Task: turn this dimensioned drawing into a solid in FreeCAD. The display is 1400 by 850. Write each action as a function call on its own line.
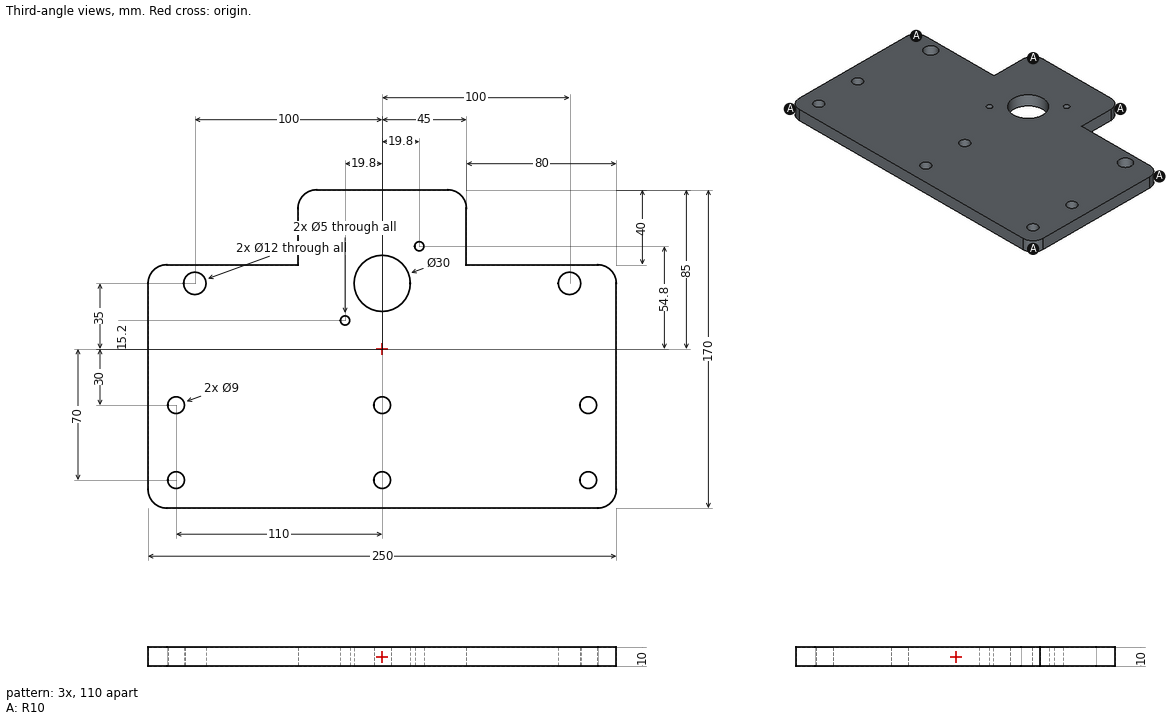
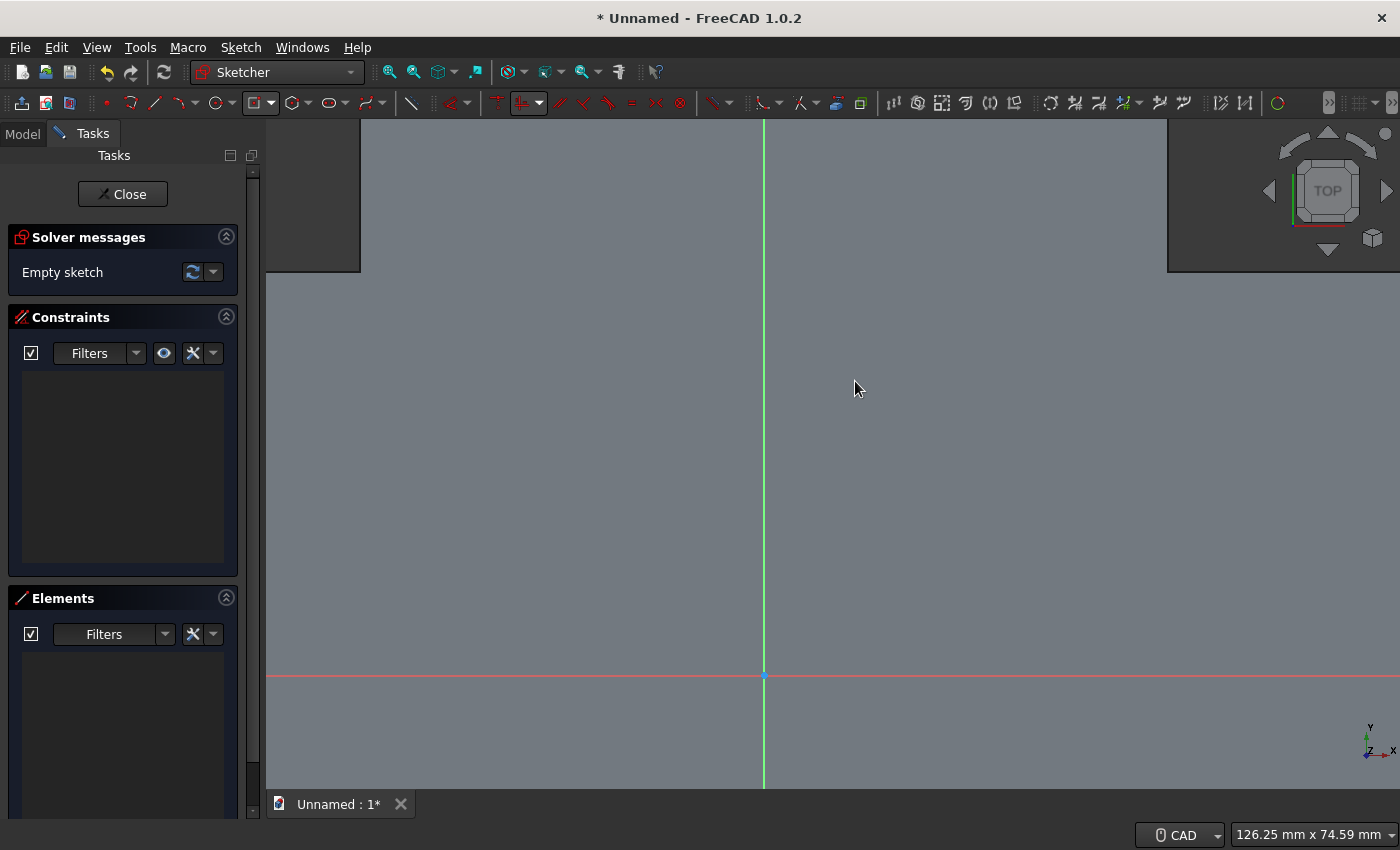
click(216, 104)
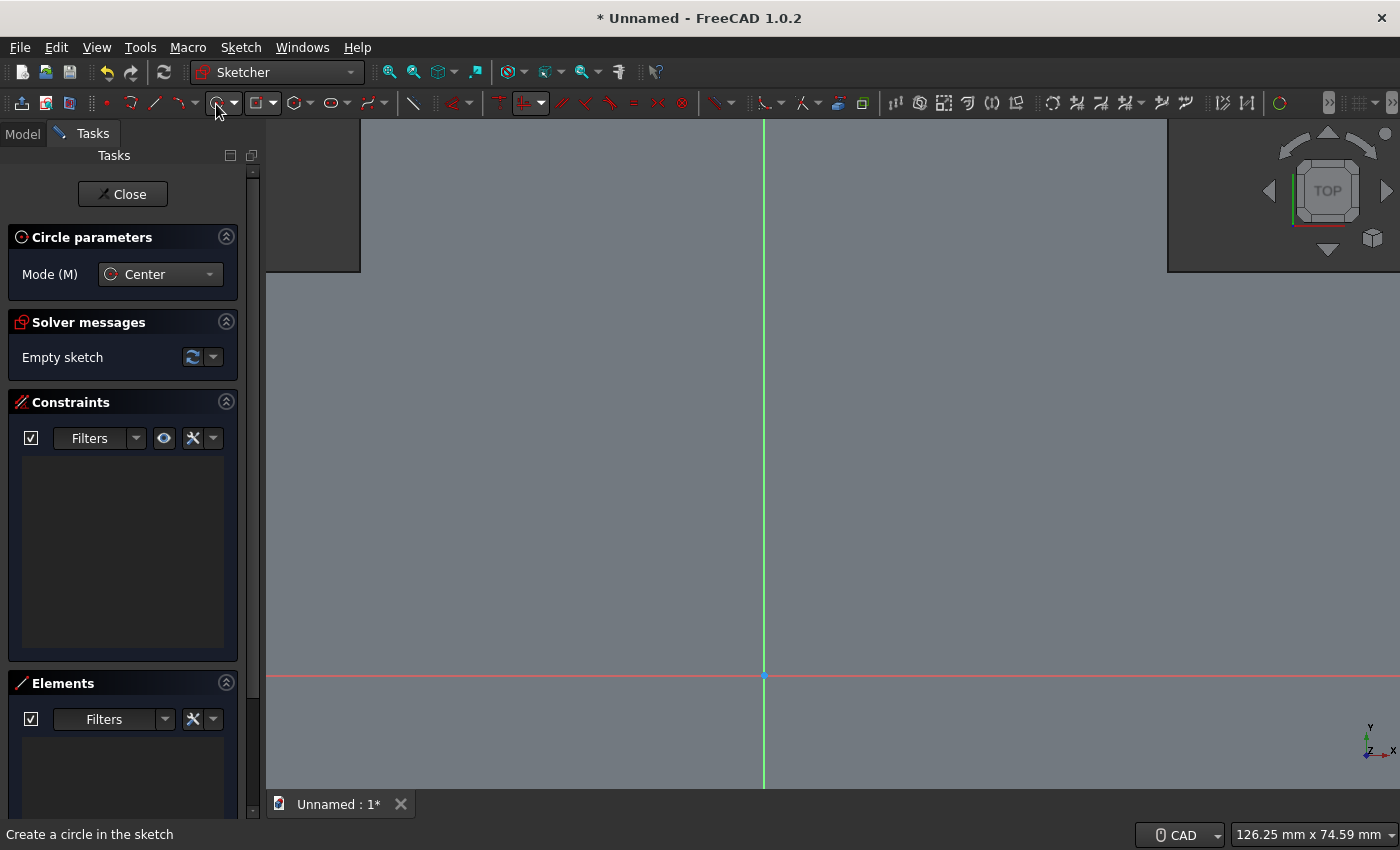
click(764, 361)
move(859, 266)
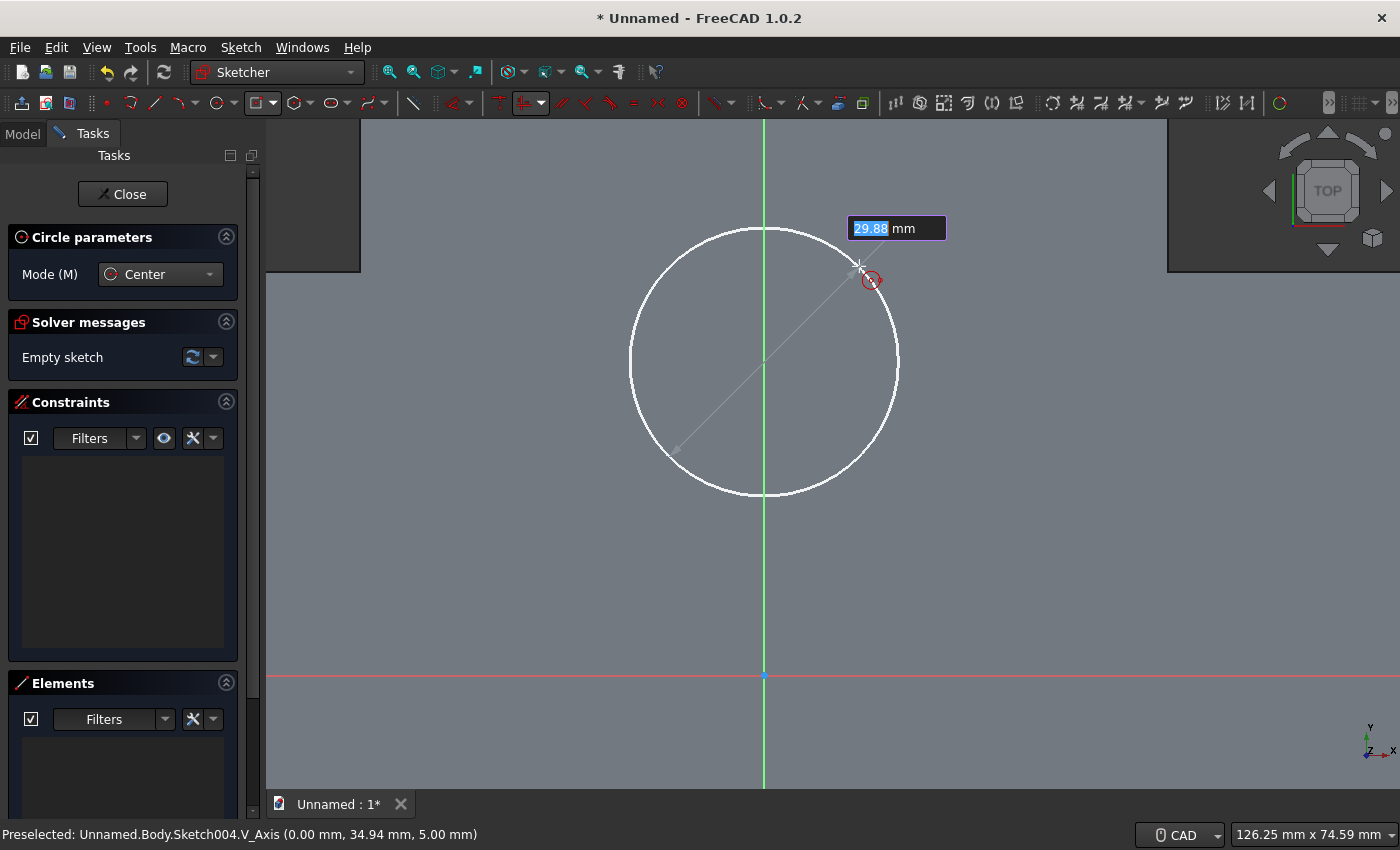
text(30)
key(Return)
key(Escape)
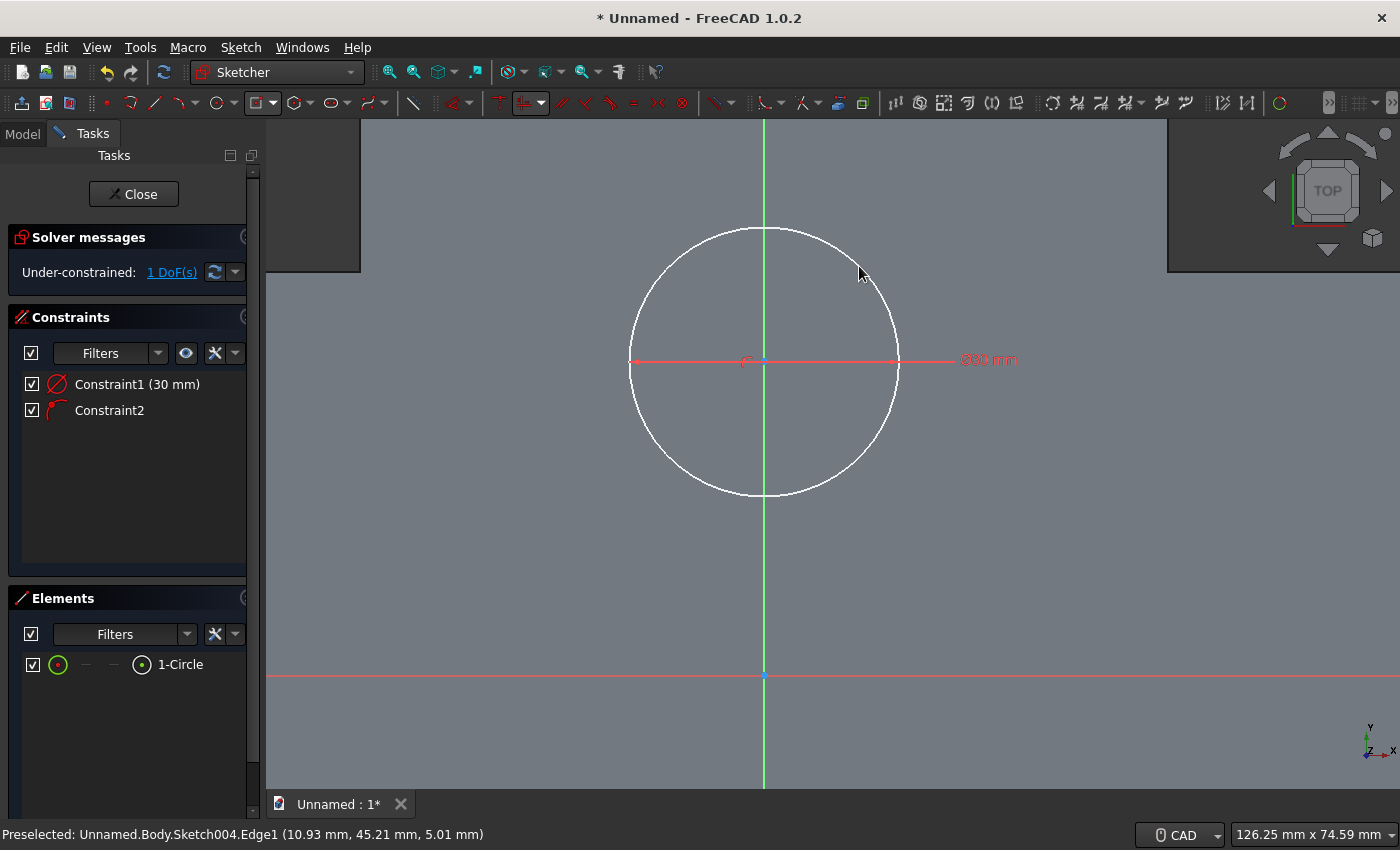
click(452, 104)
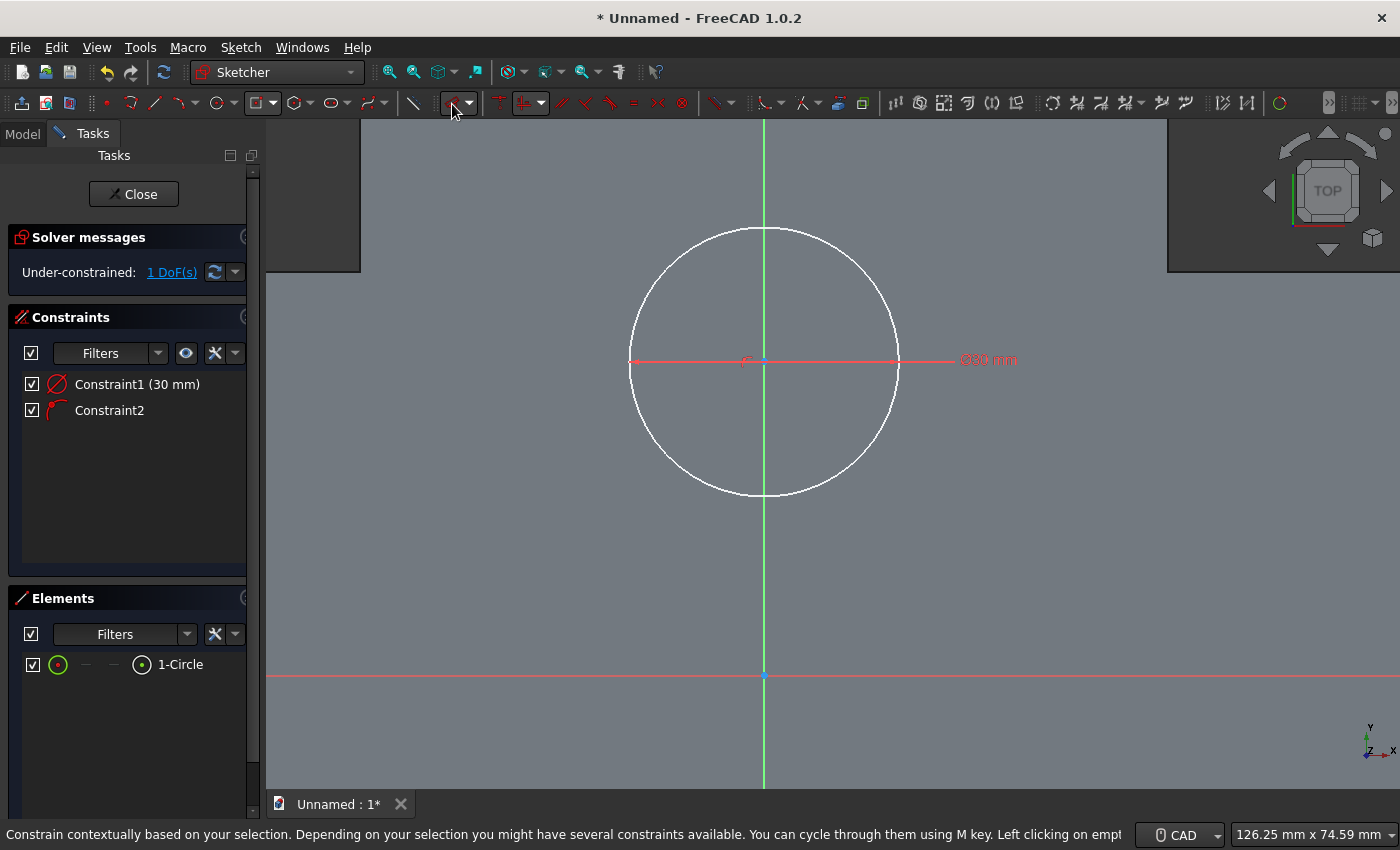
click(764, 362)
click(798, 519)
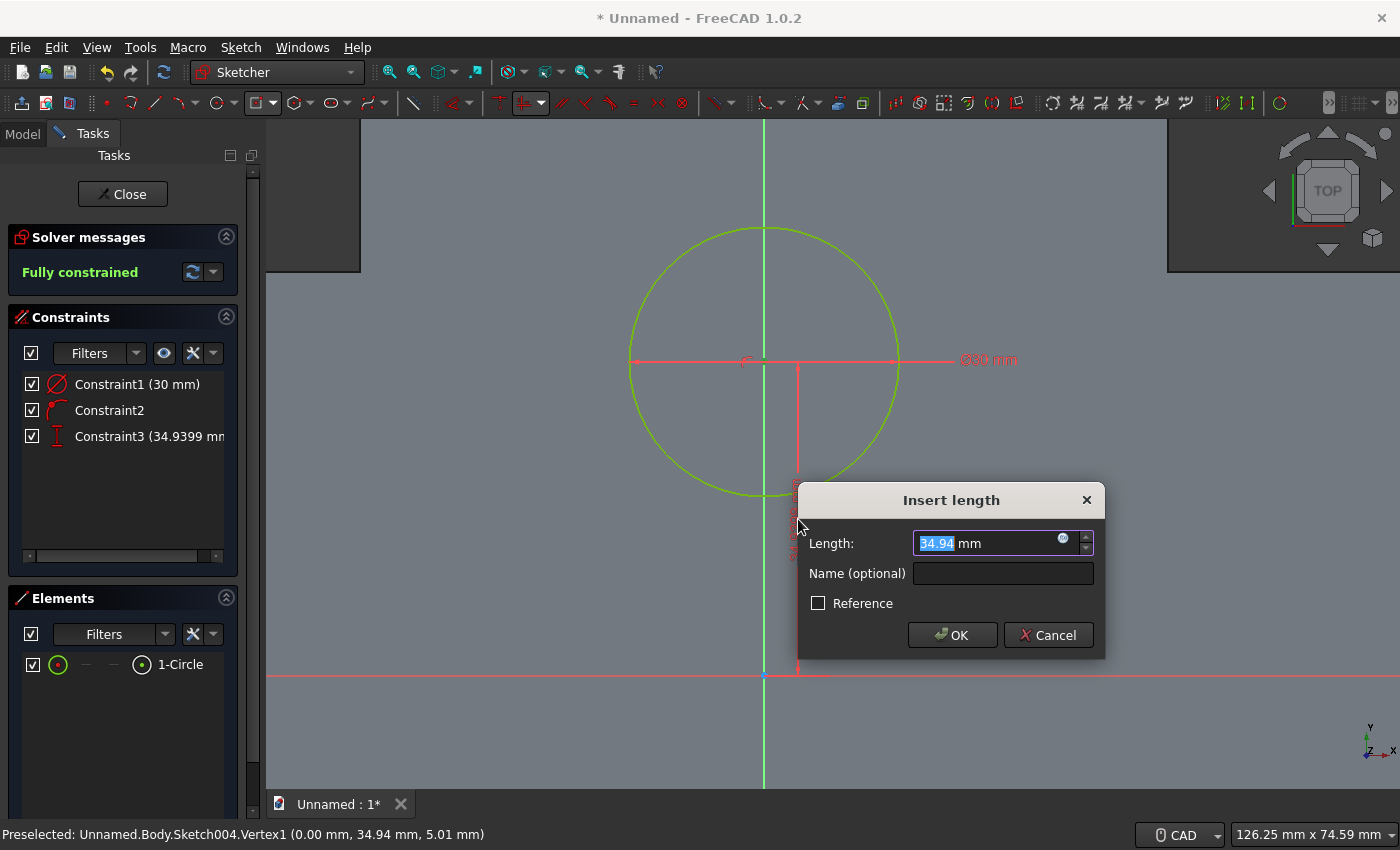
text(35)
key(Return)
key(Escape)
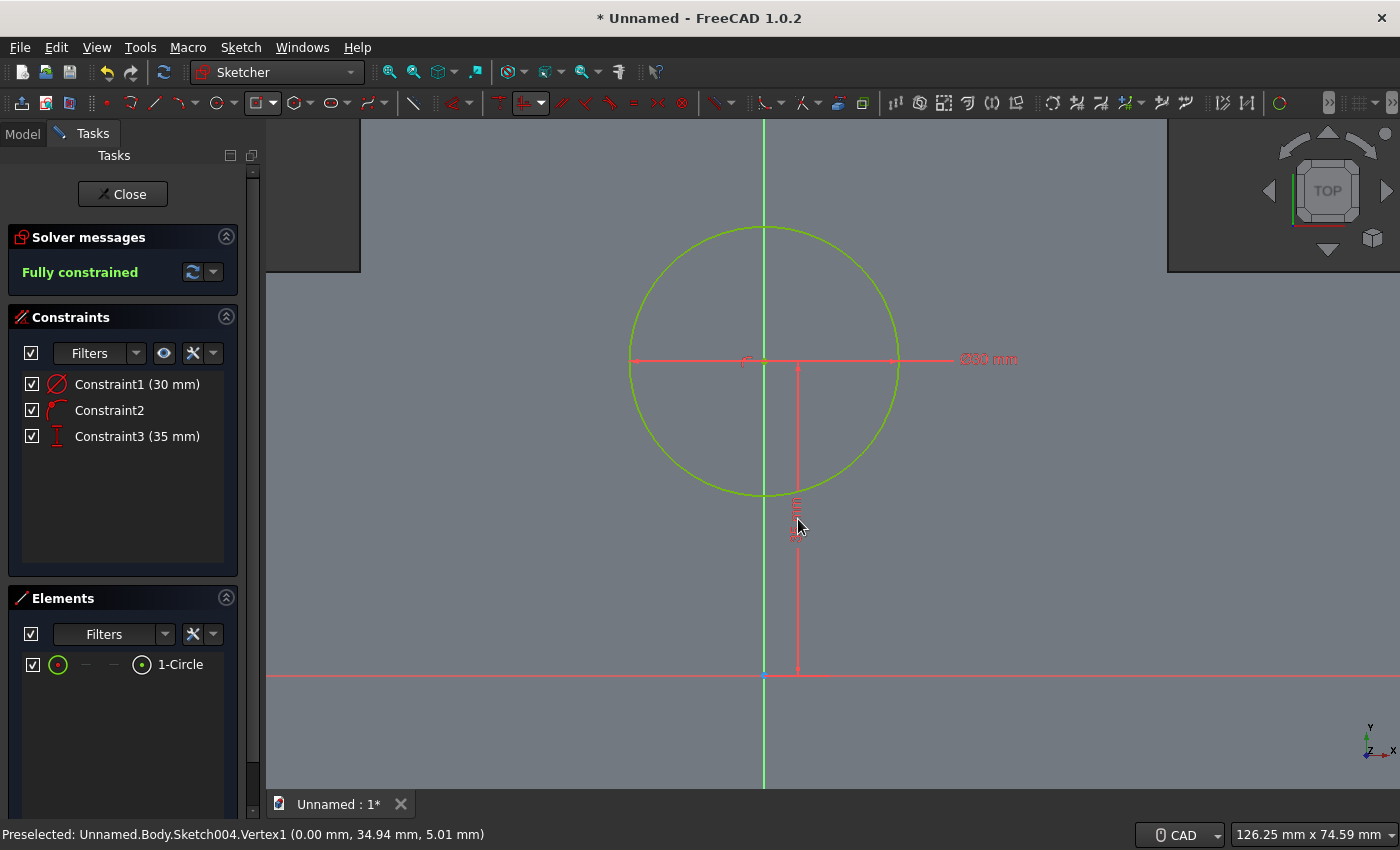
click(123, 194)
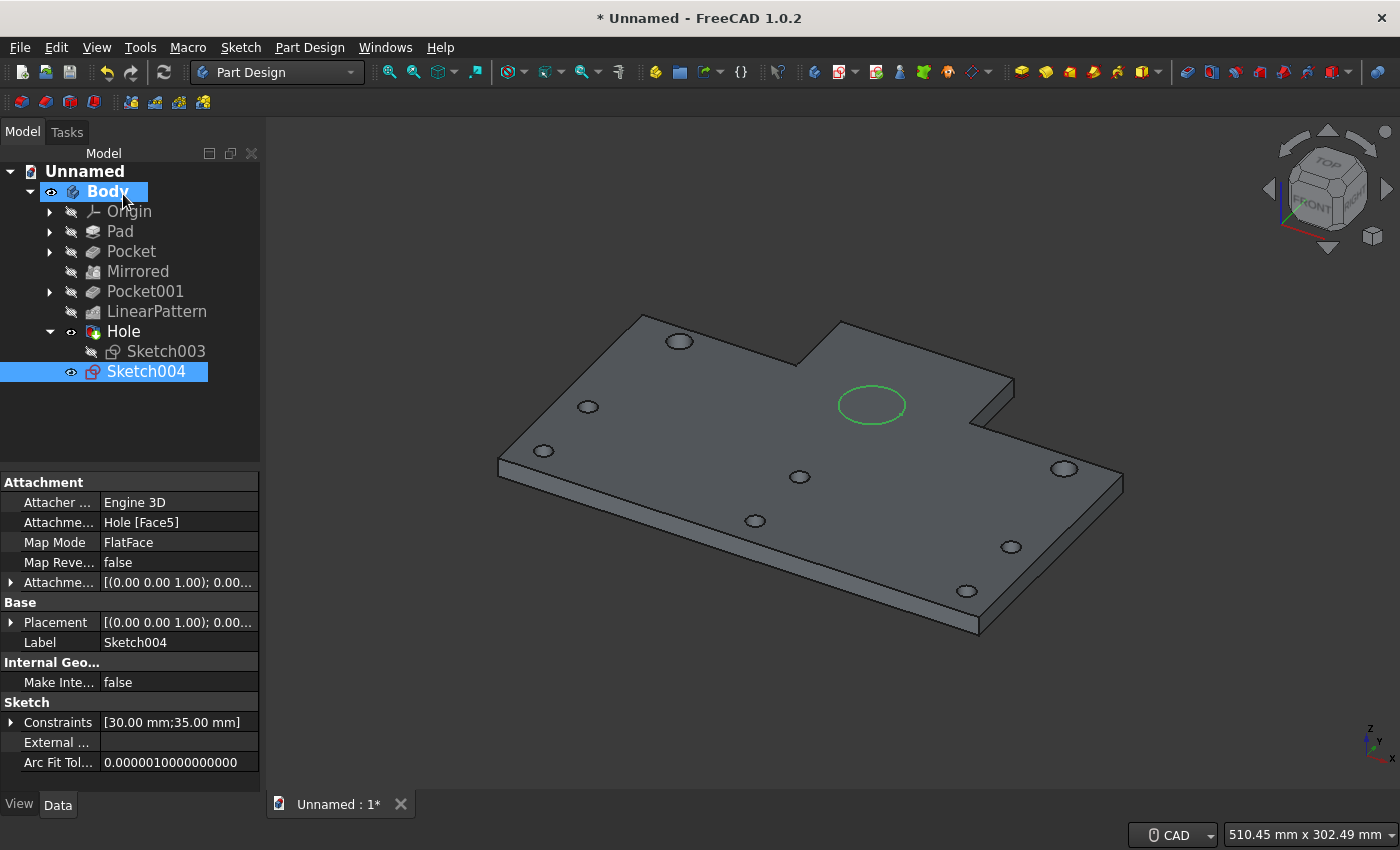
click(1188, 72)